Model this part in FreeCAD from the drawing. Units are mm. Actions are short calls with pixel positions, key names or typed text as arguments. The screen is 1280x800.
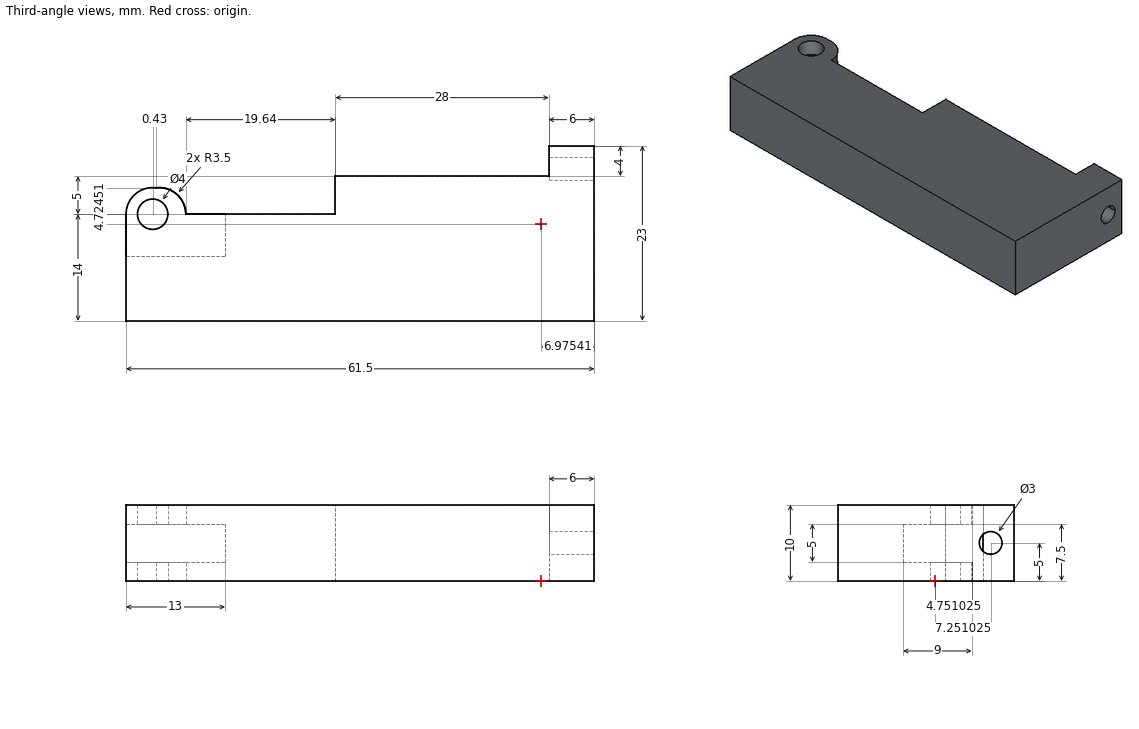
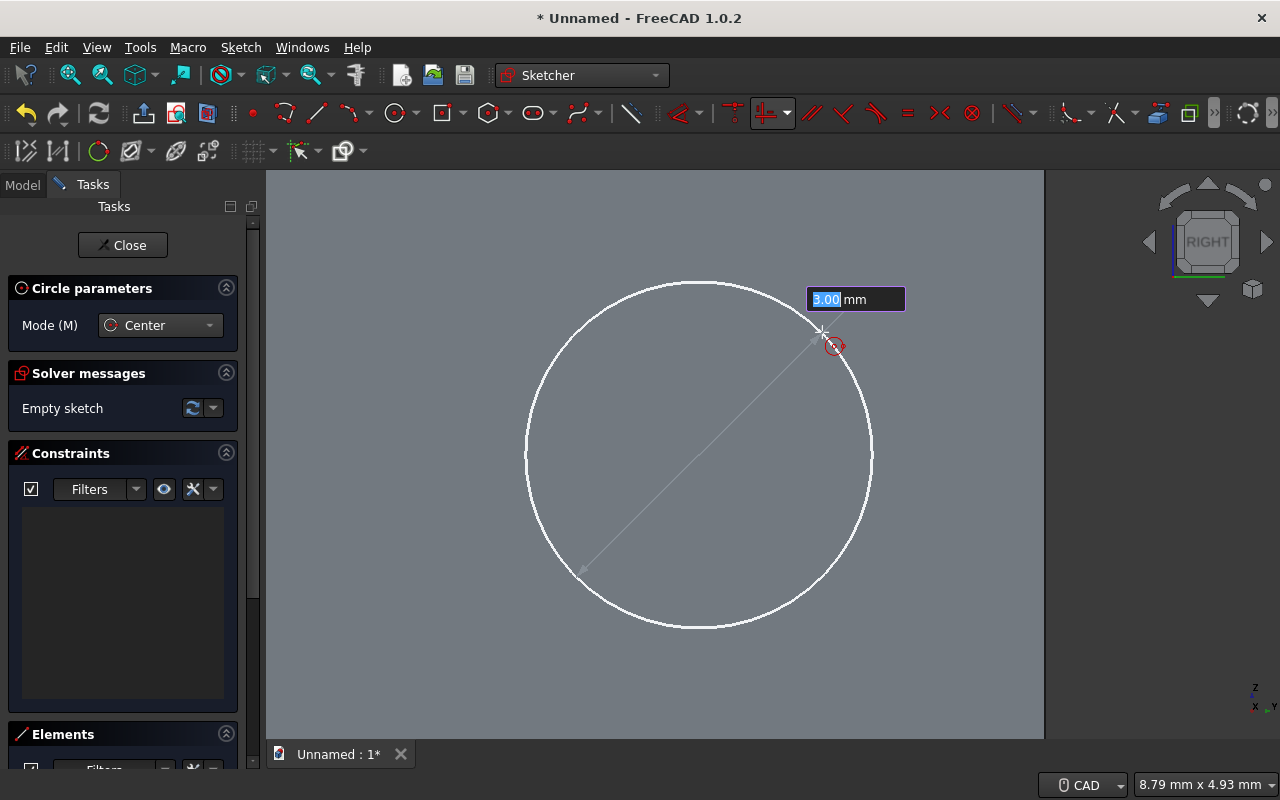
text(3)
key(Return)
key(Escape)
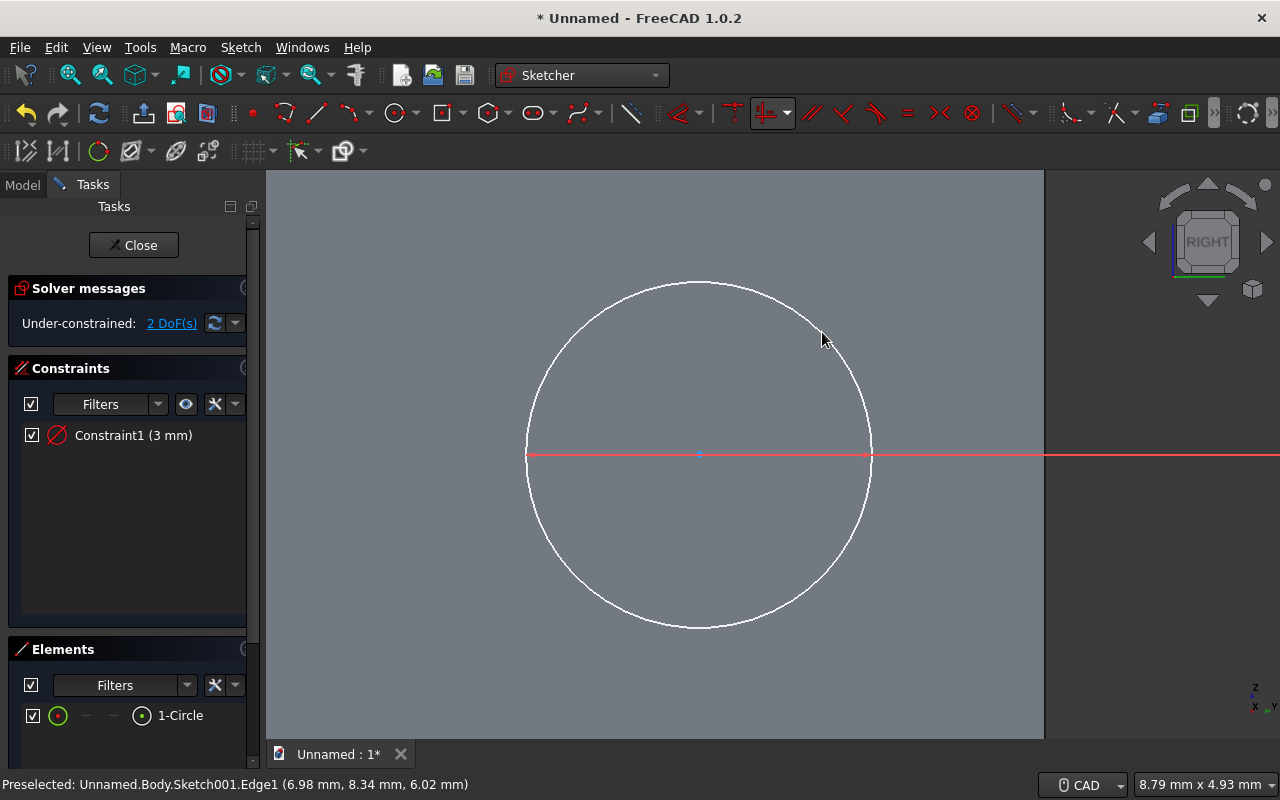
key(d)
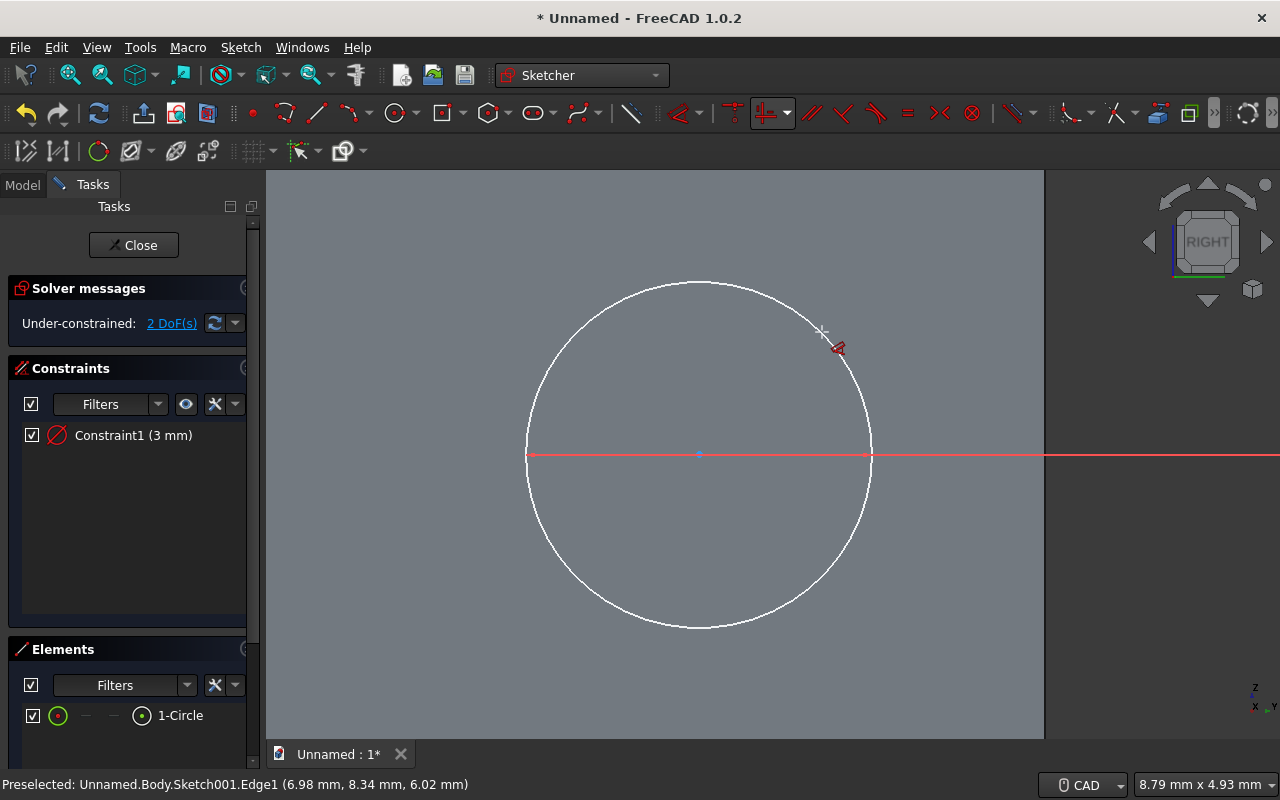
click(699, 455)
click(733, 583)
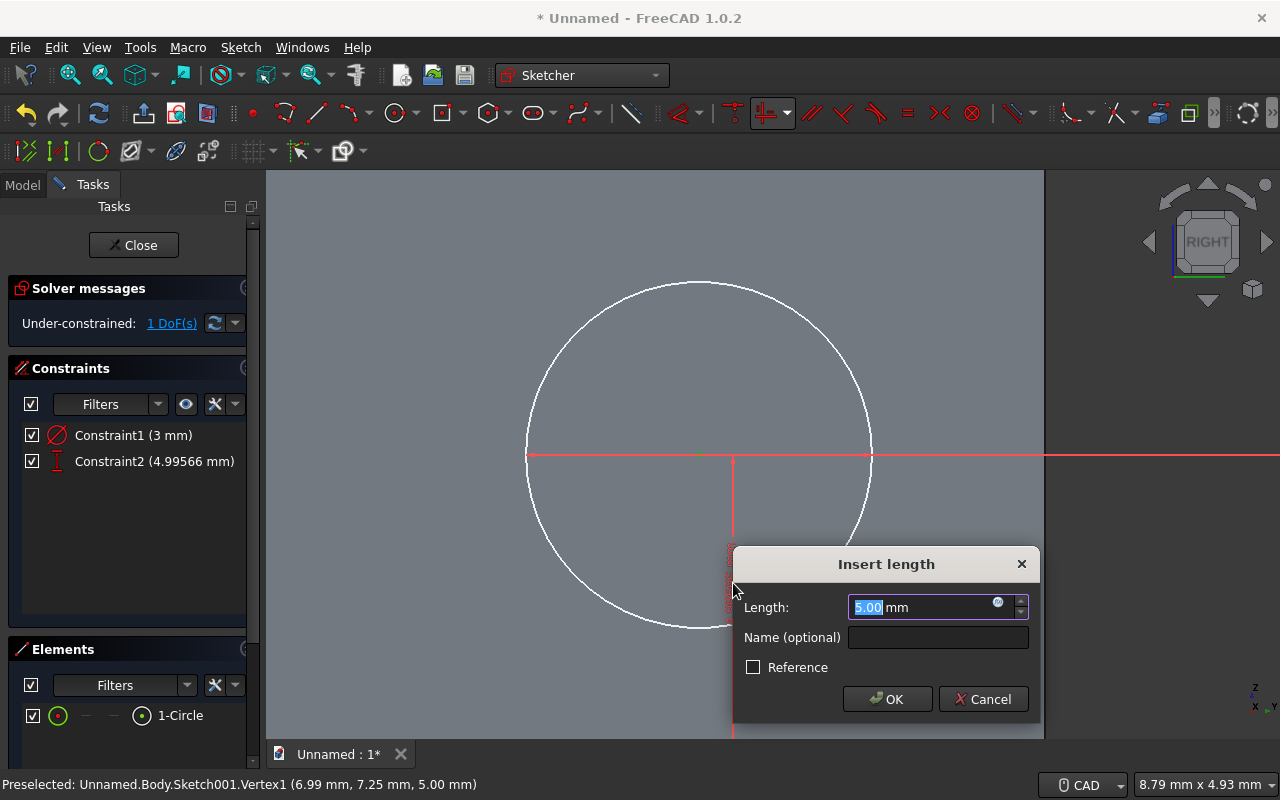
text(5)
key(Return)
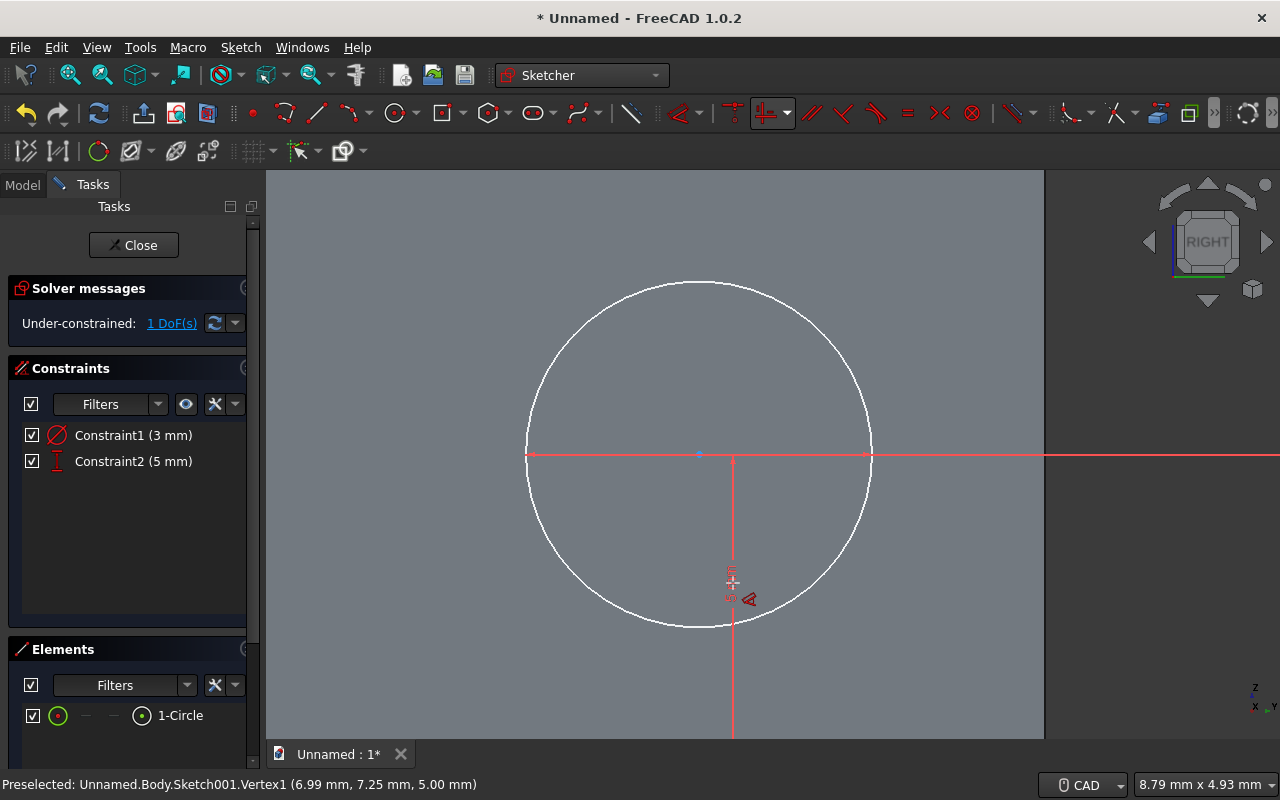
click(699, 454)
click(496, 420)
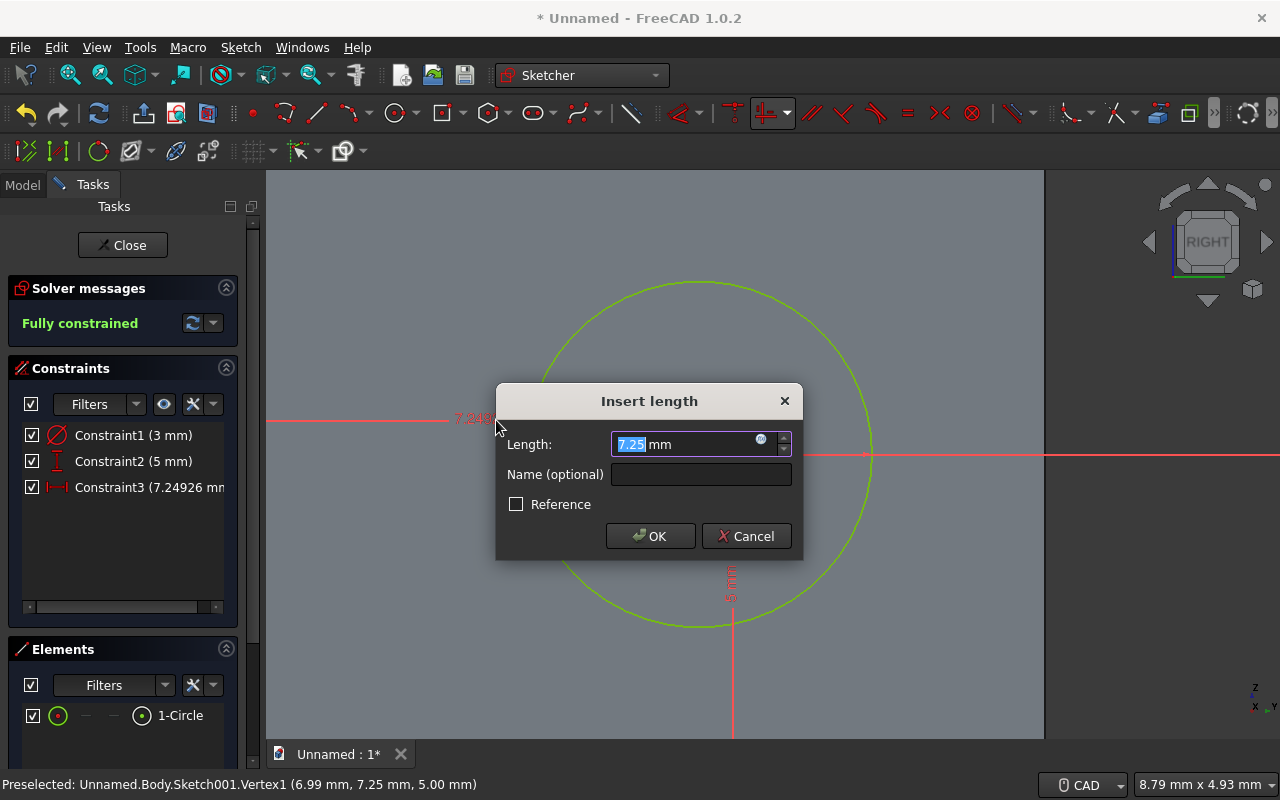
text(7.251025)
key(Return)
key(Escape)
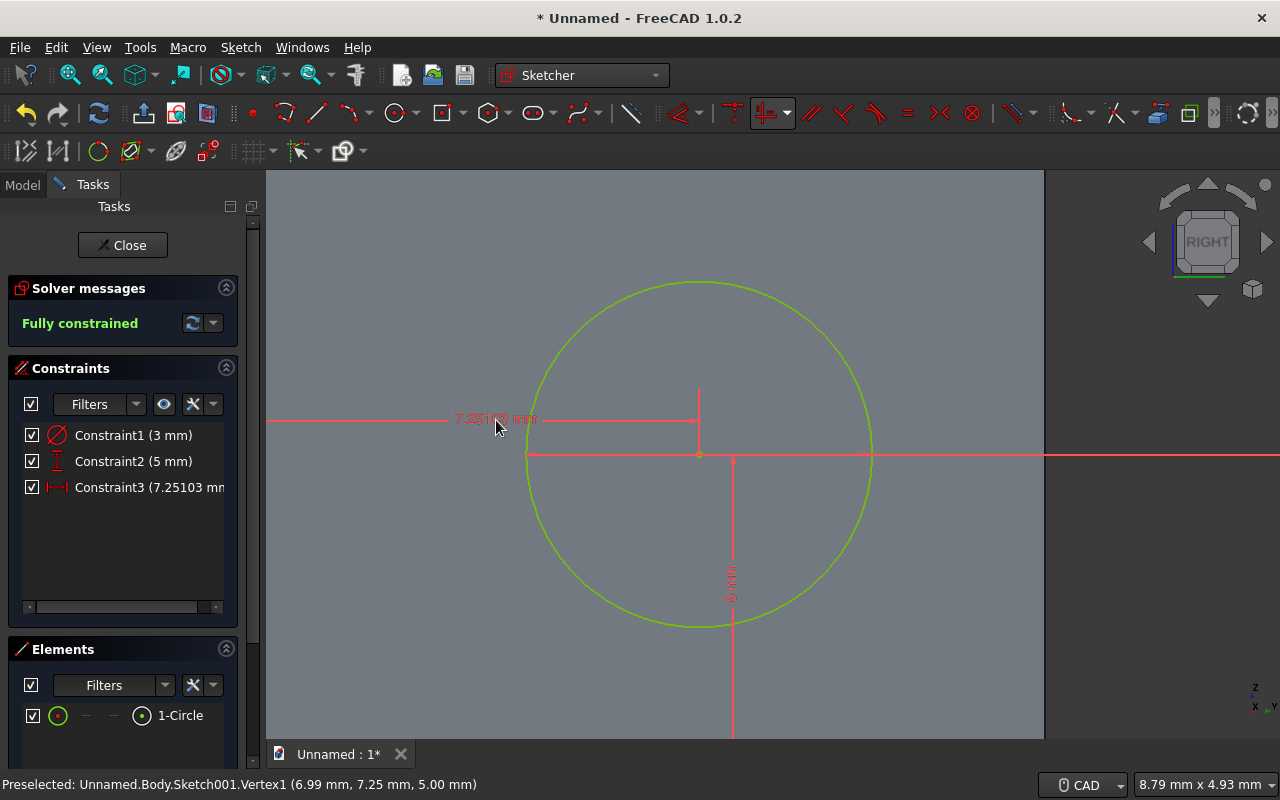
click(123, 245)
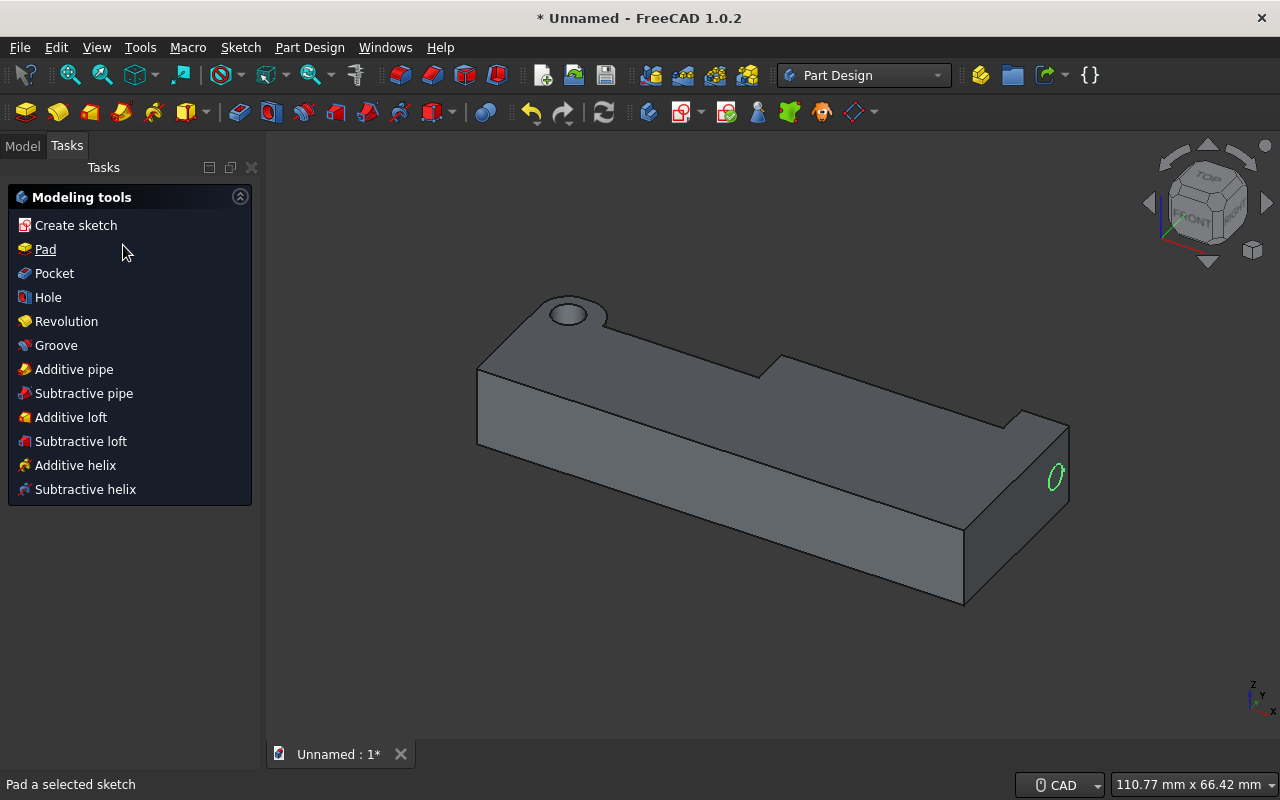
click(240, 112)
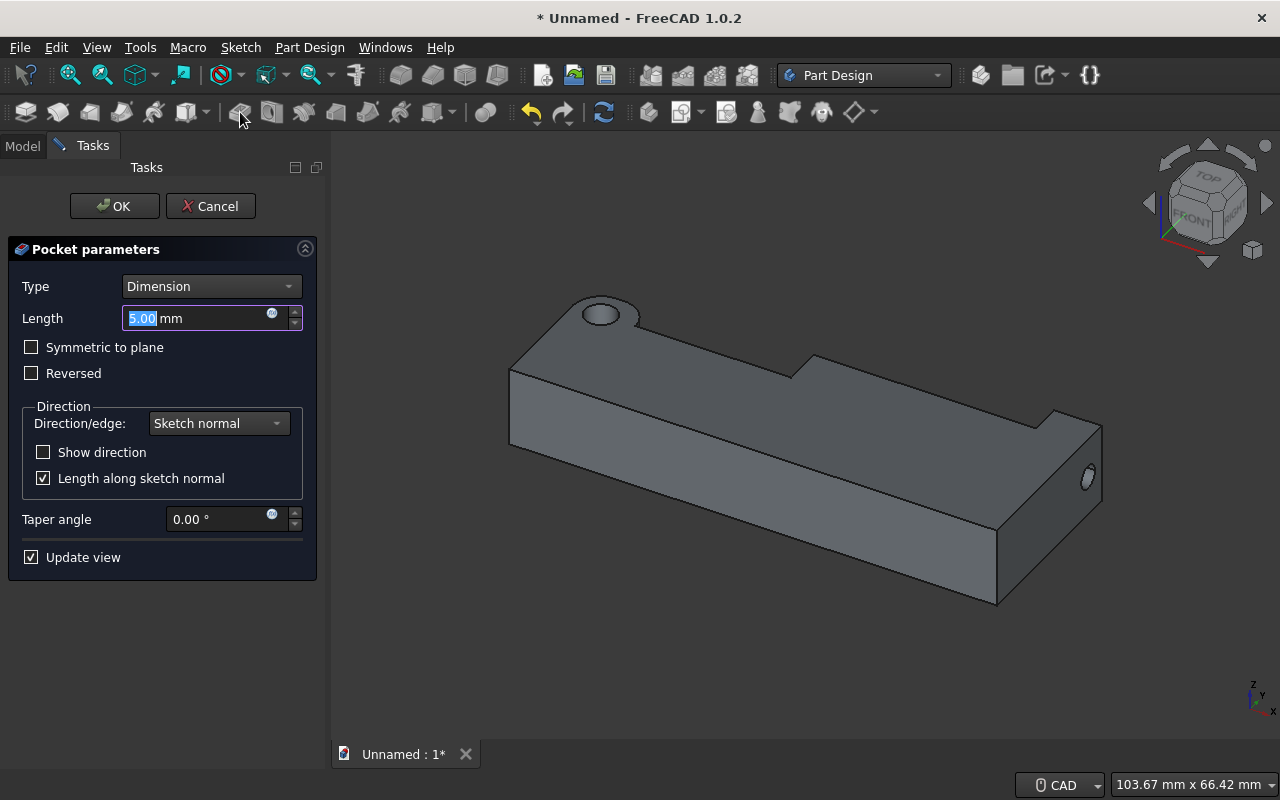
text(6)
key(Tab)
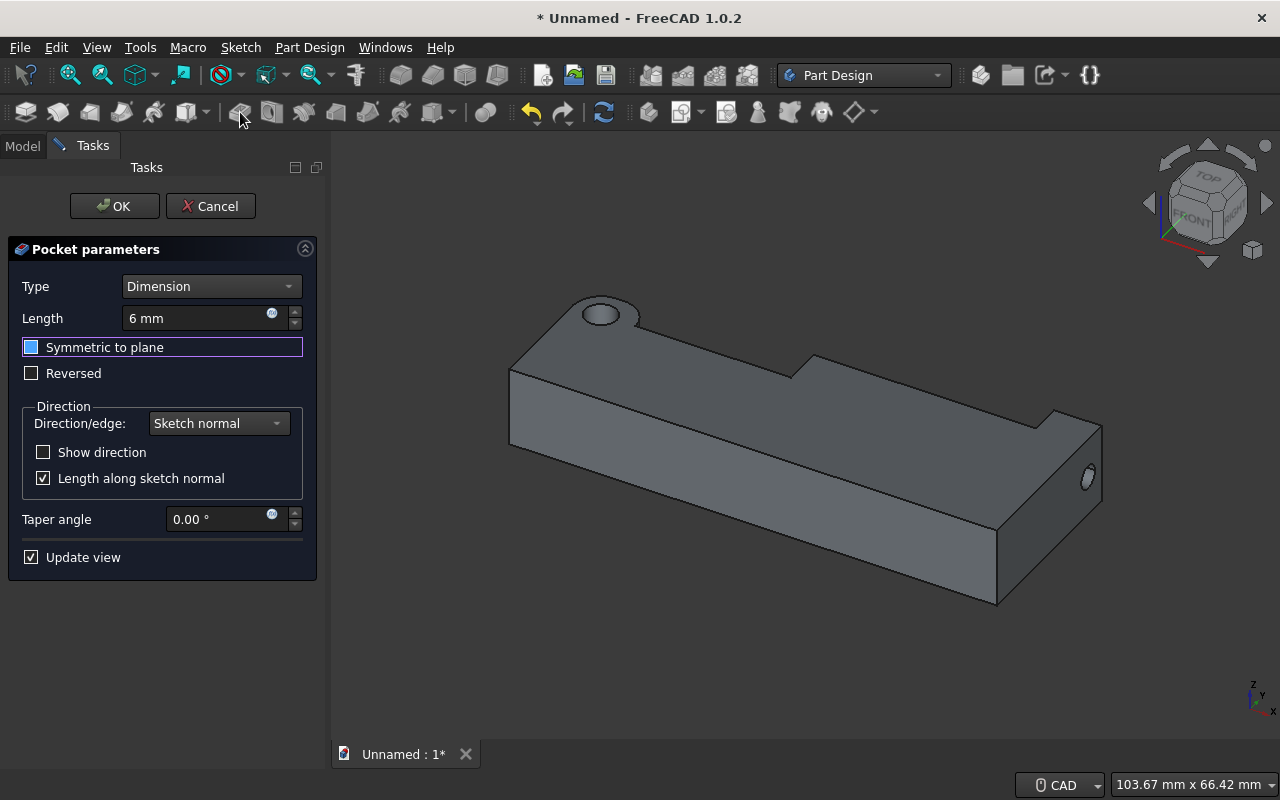
click(115, 206)